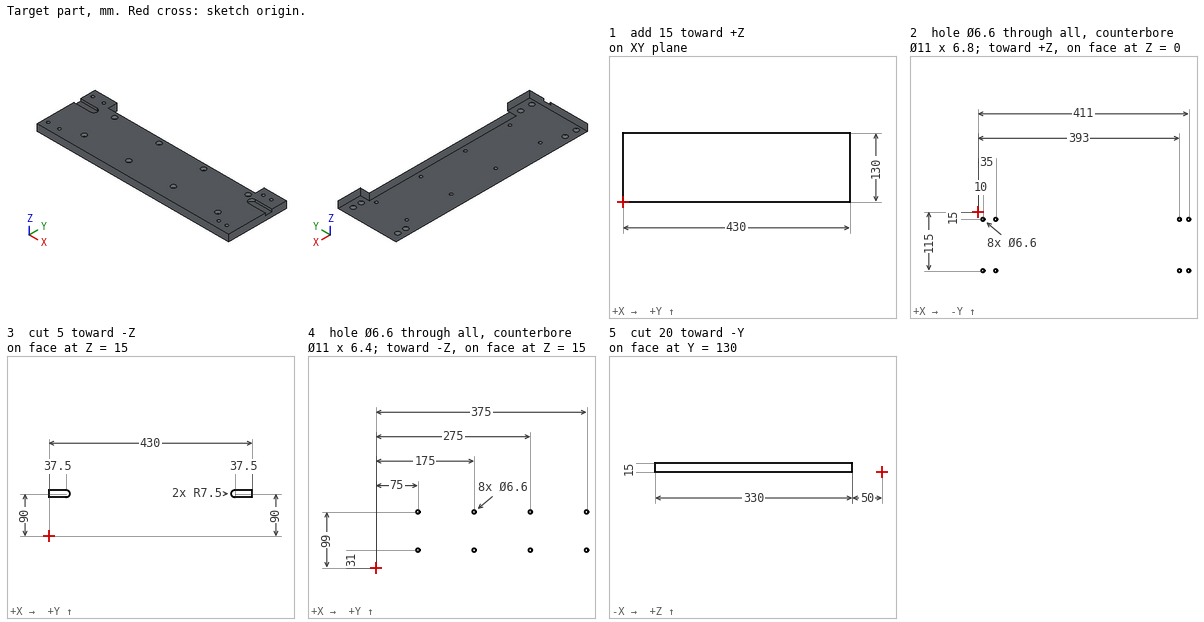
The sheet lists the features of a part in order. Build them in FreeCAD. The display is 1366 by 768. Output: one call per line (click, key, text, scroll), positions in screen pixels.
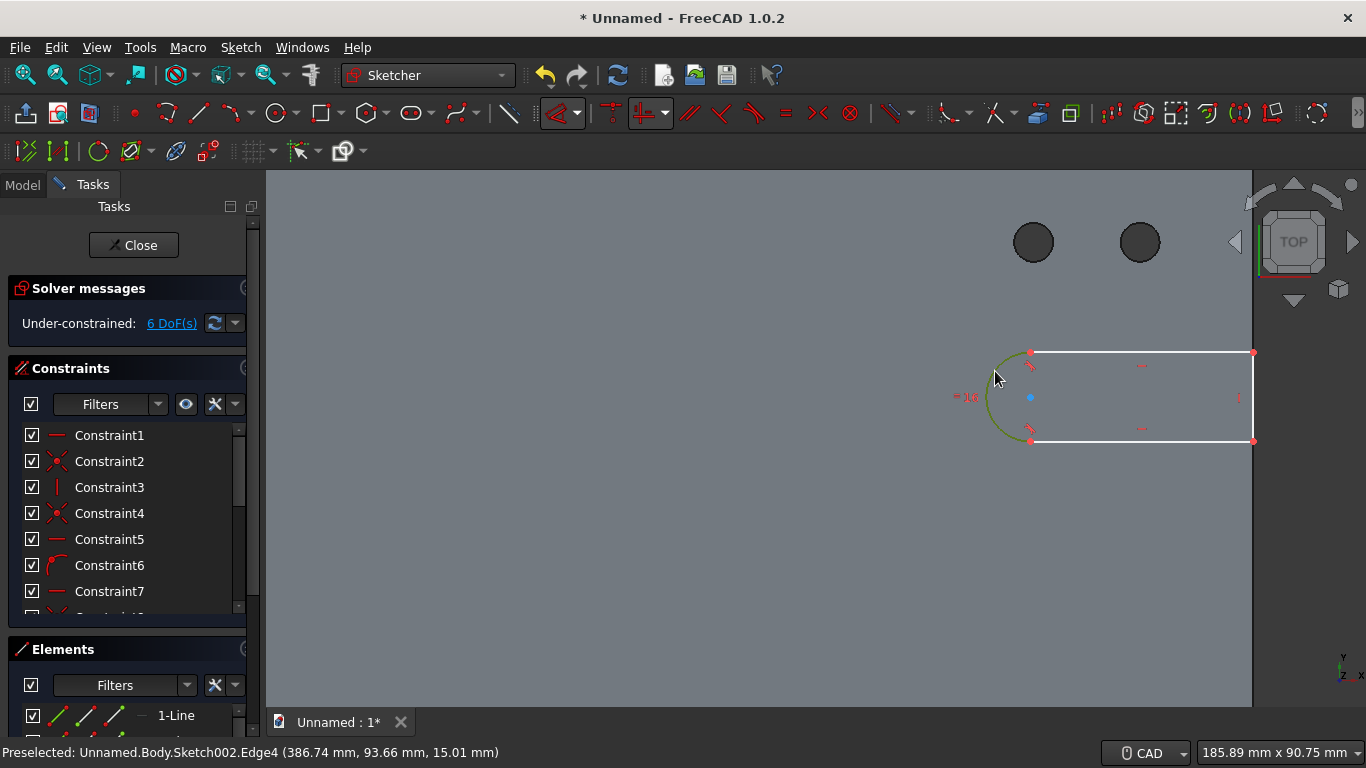
click(580, 114)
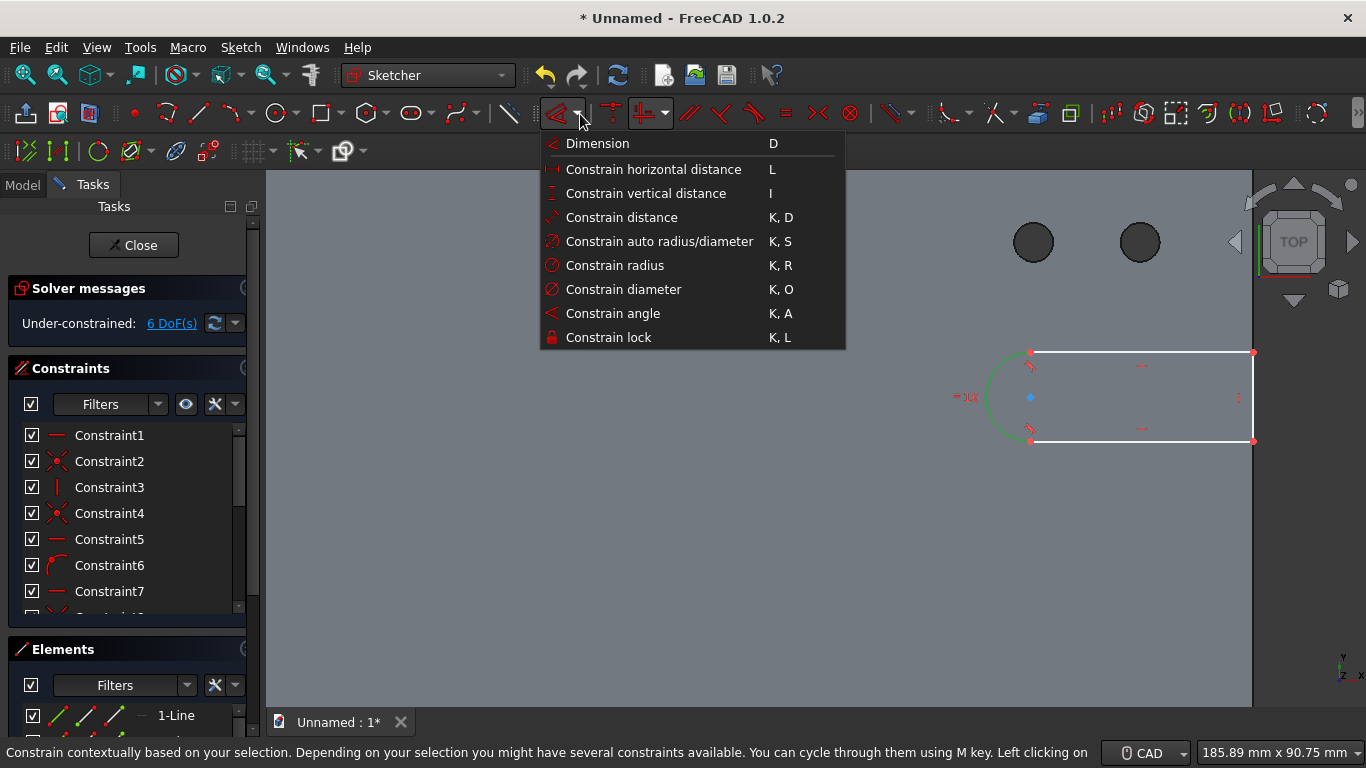
click(693, 265)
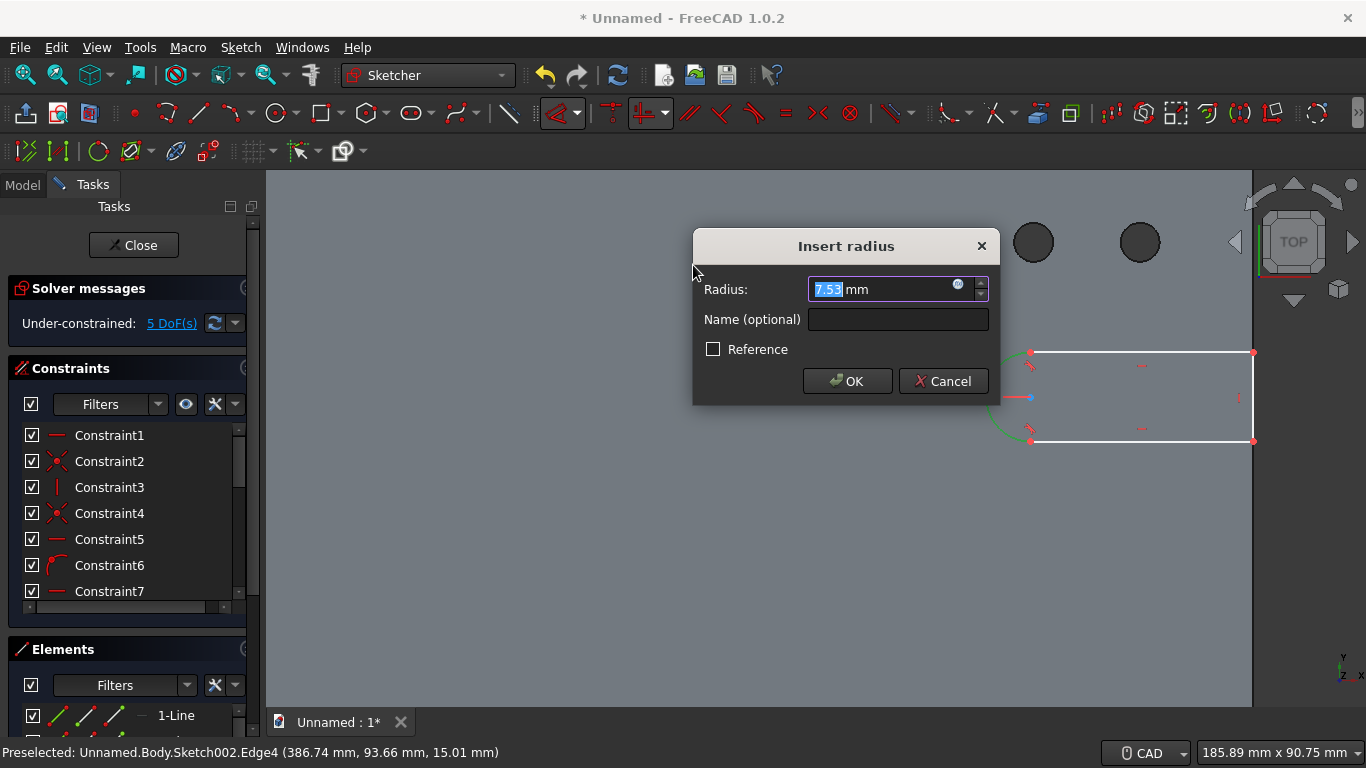
text(7.5)
key(Return)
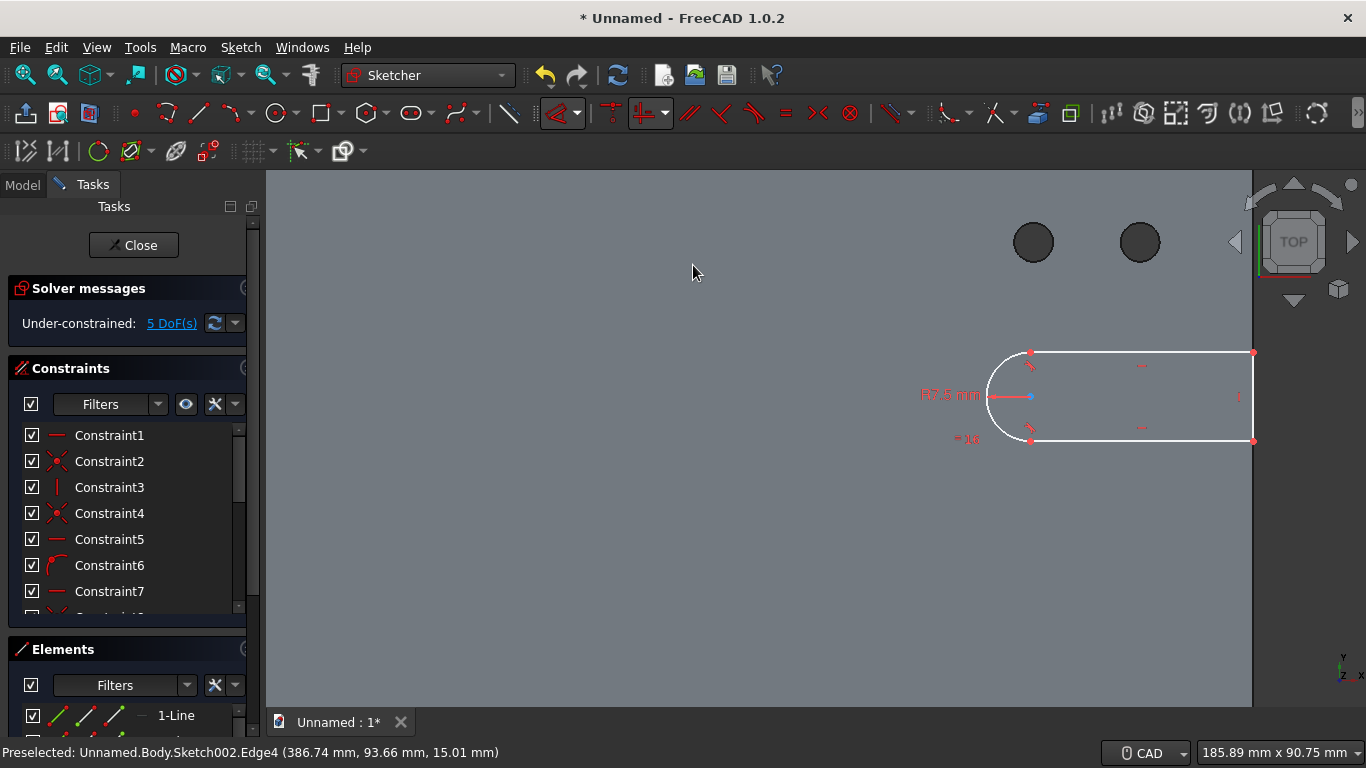
scroll(999, 374, down, 7)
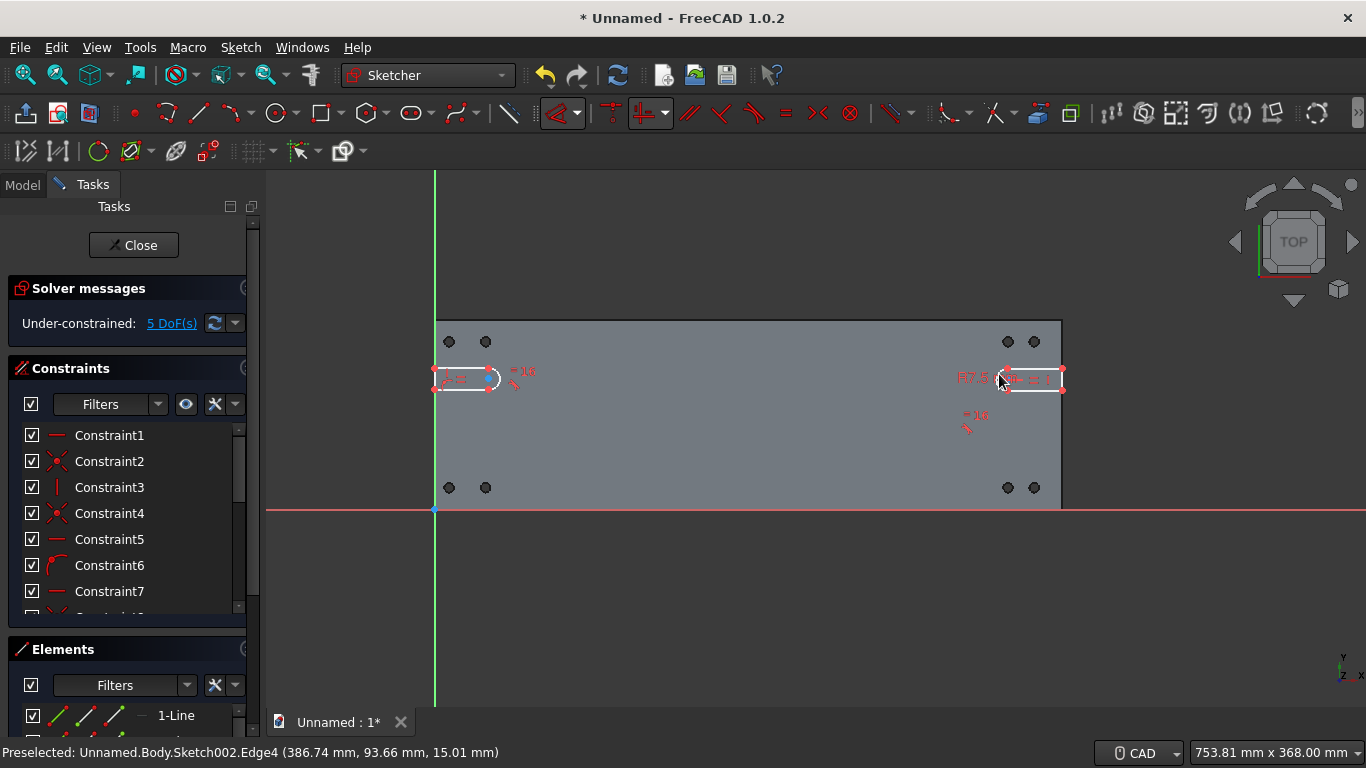
click(1007, 380)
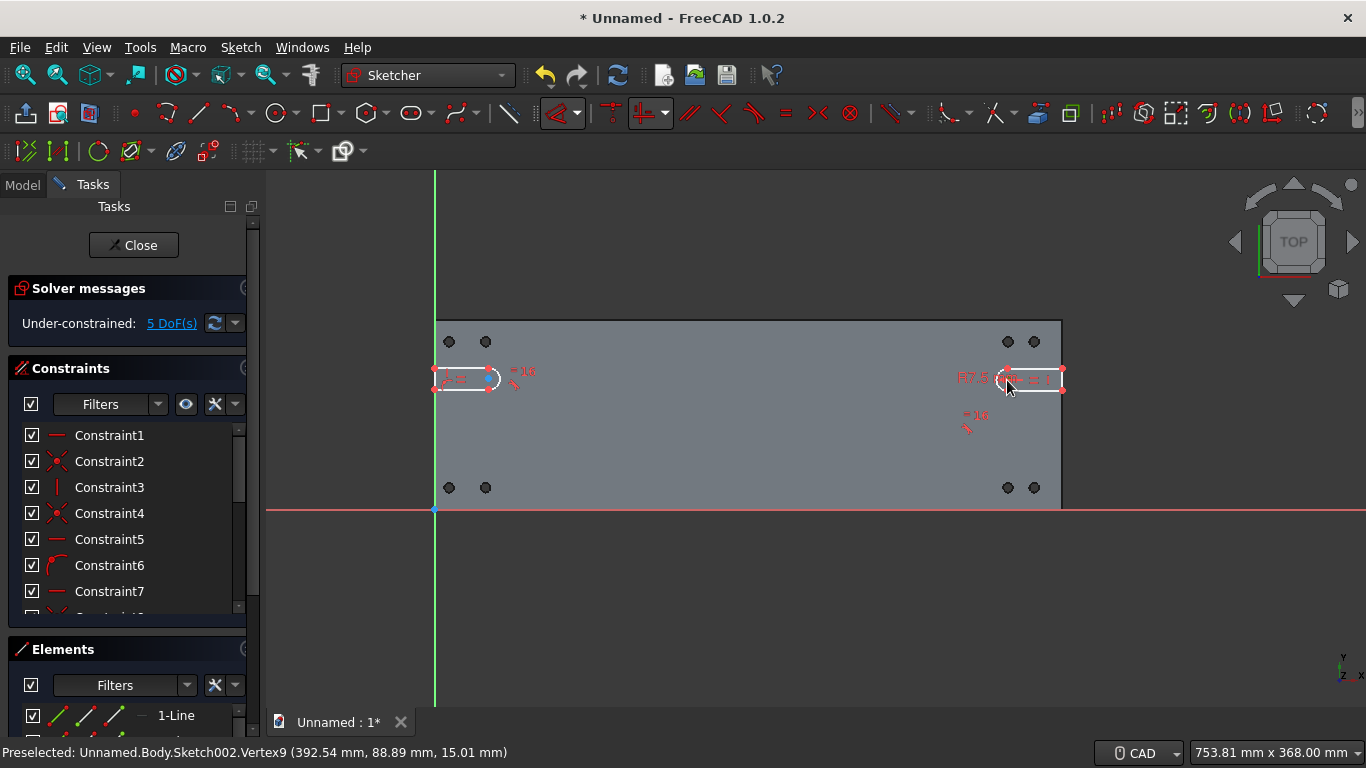
click(580, 114)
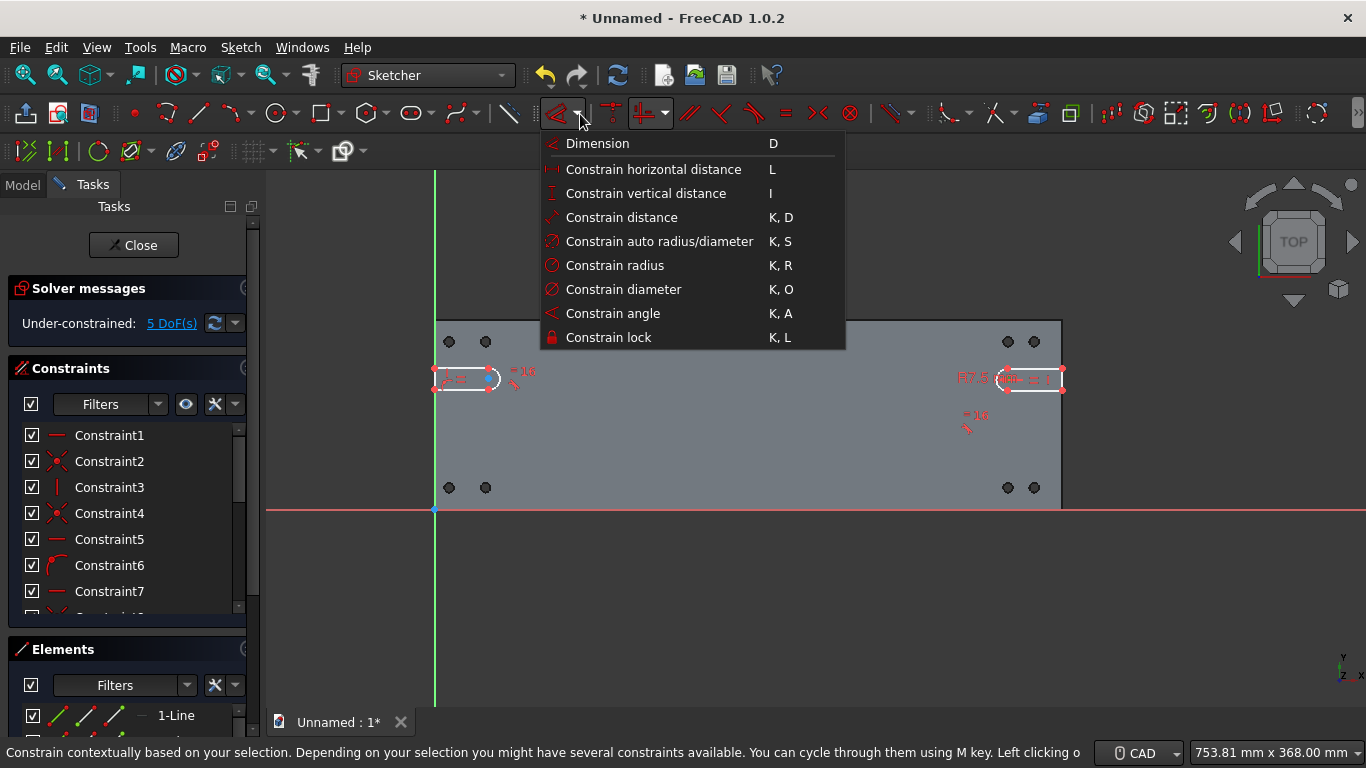
click(693, 193)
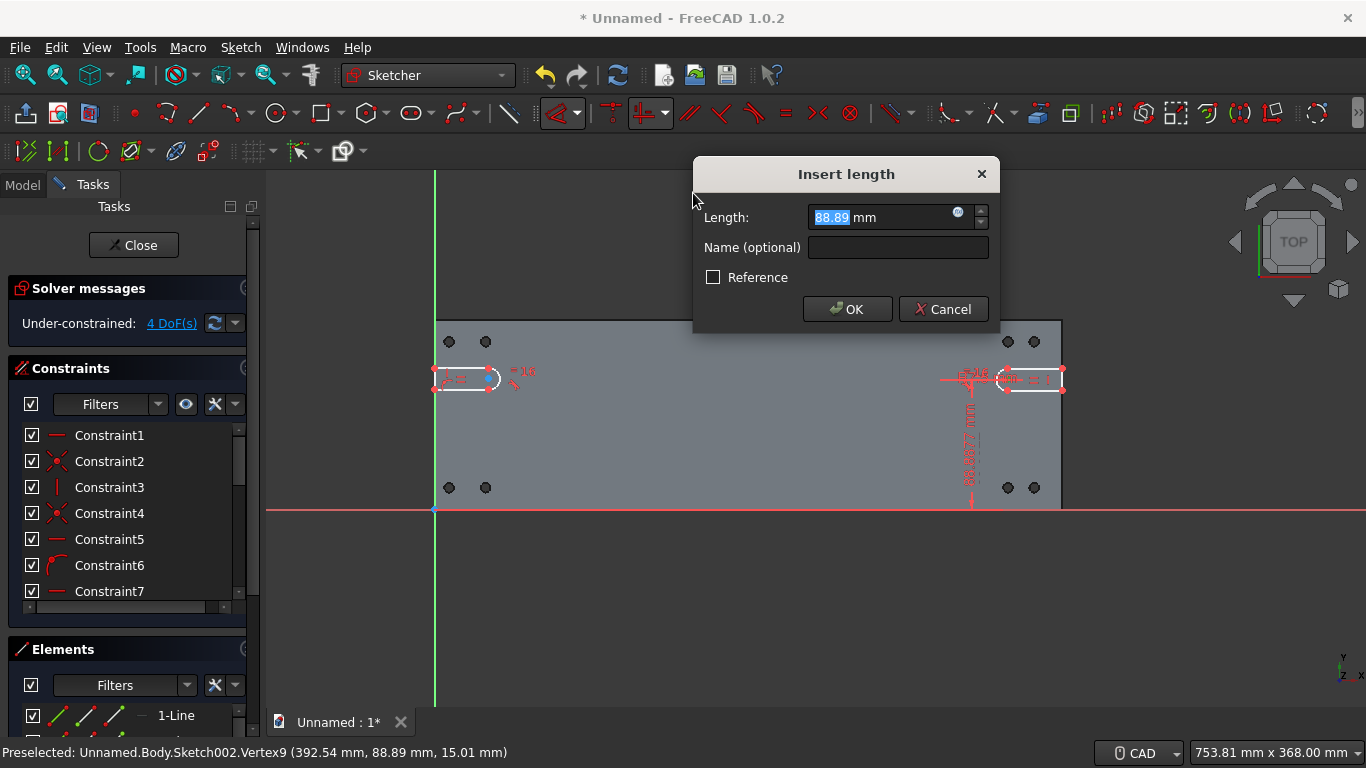
text(90)
key(Return)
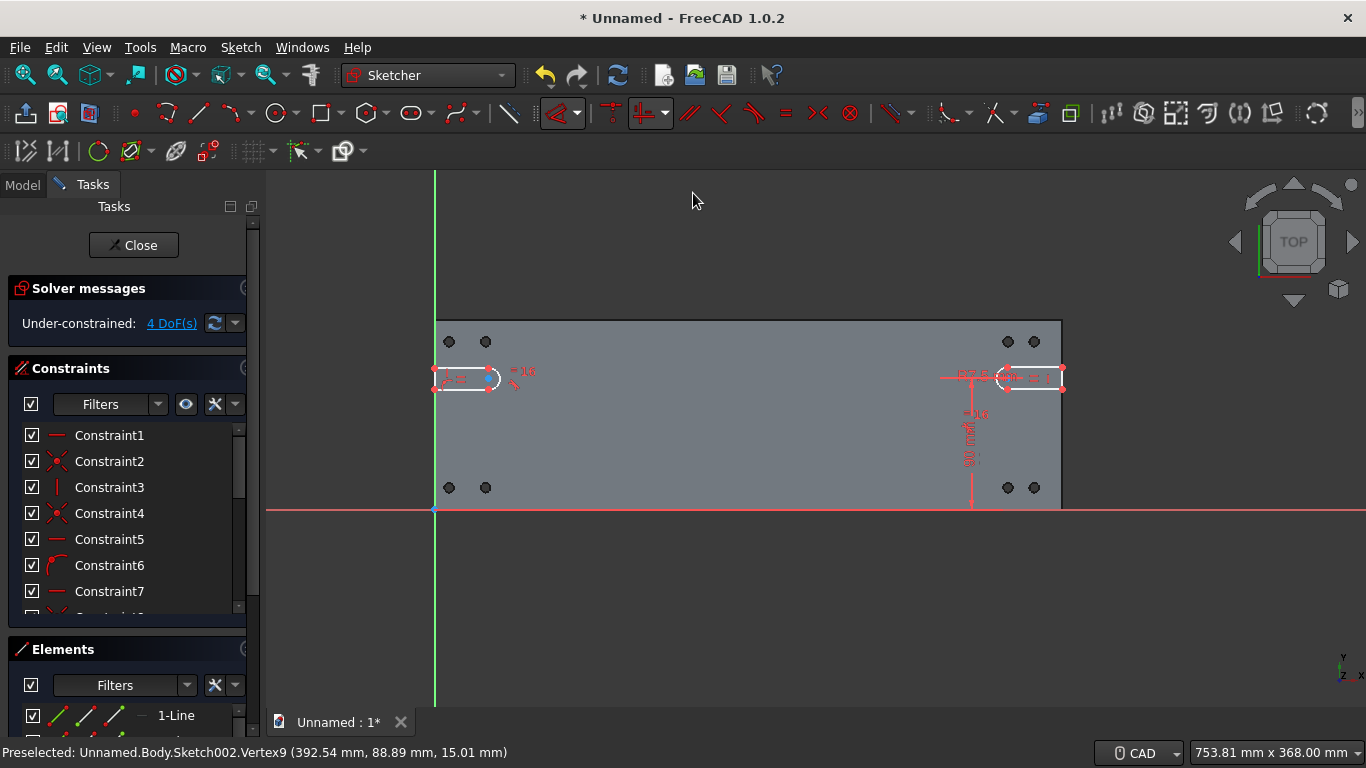
click(489, 379)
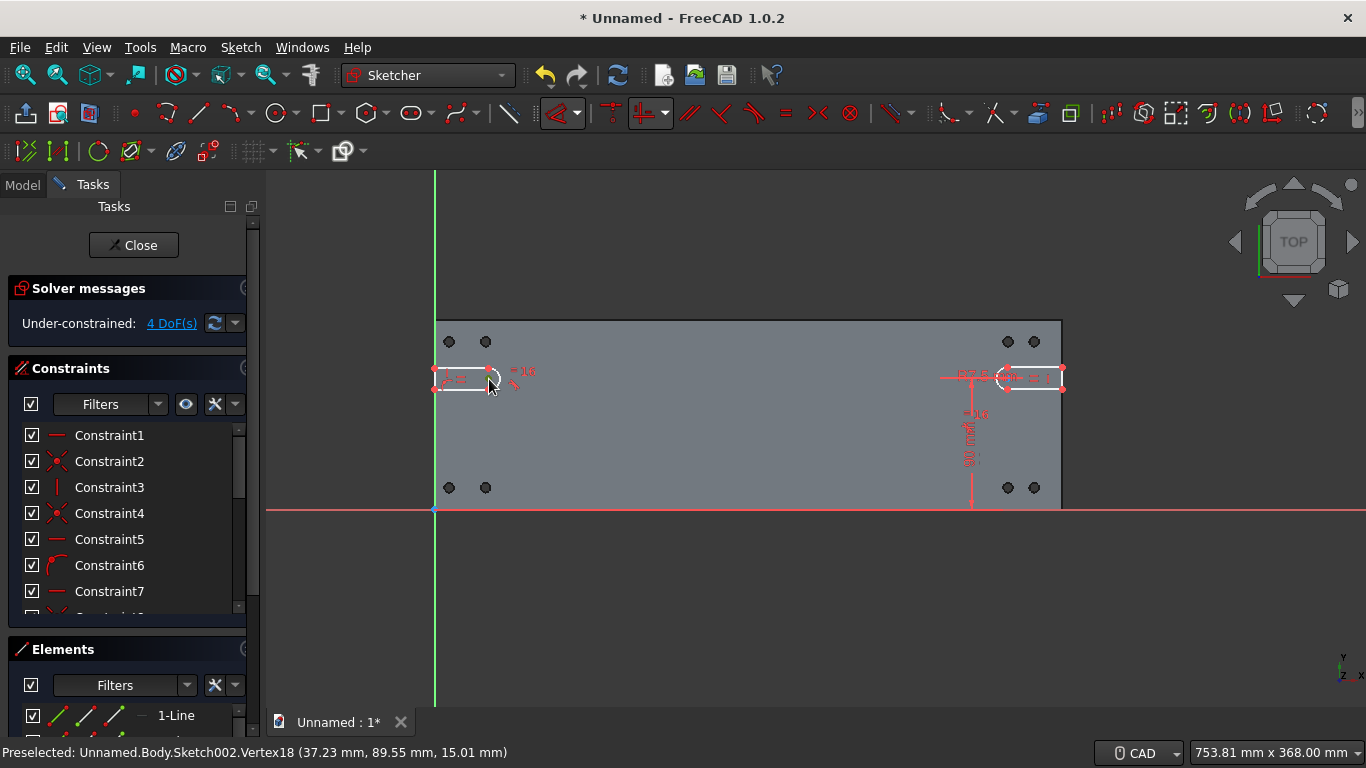
key(i)